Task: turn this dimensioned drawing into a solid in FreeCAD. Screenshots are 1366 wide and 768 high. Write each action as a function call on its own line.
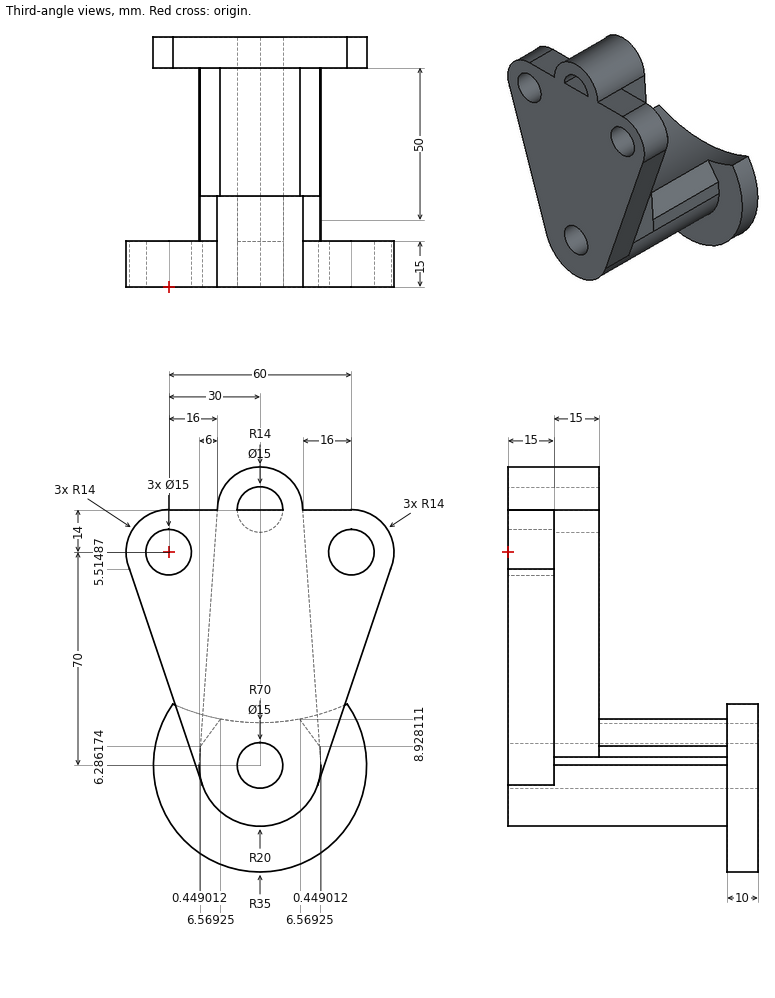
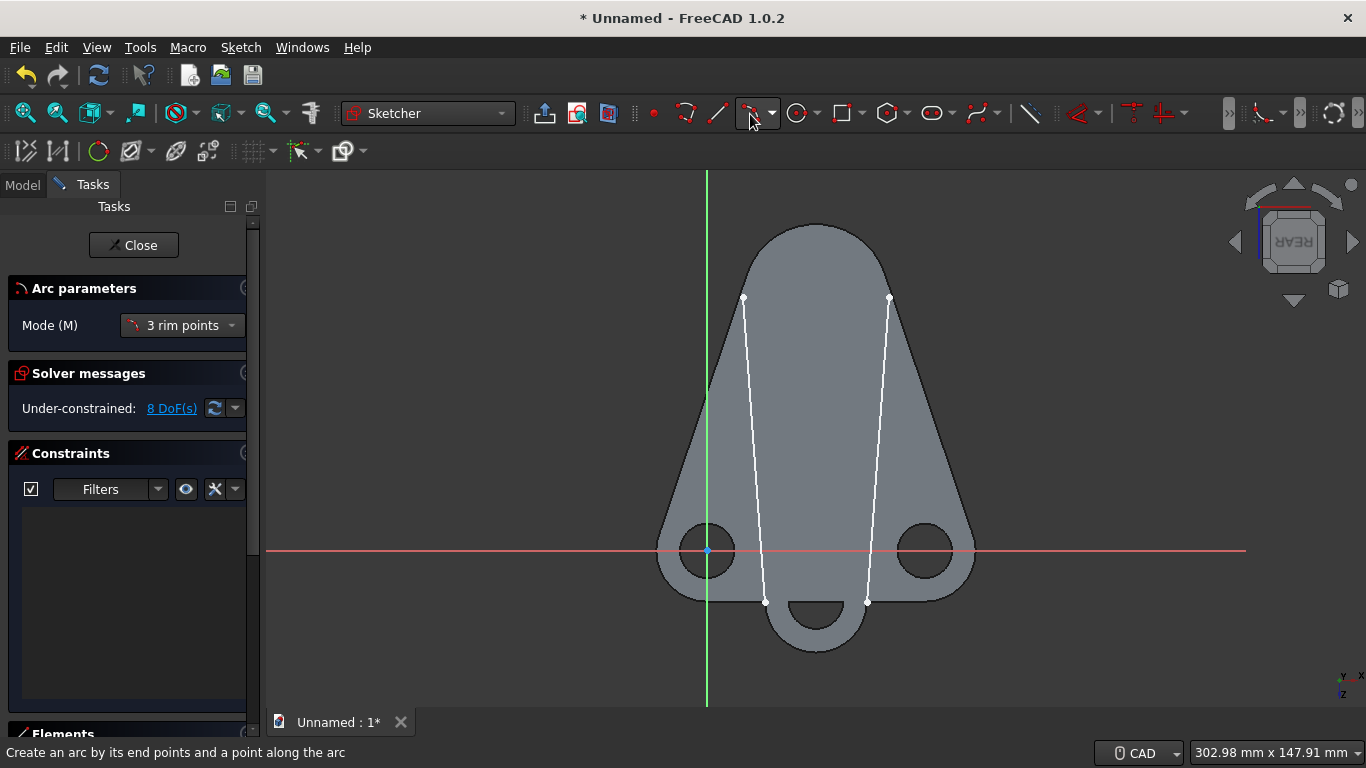
click(765, 603)
click(867, 603)
click(816, 653)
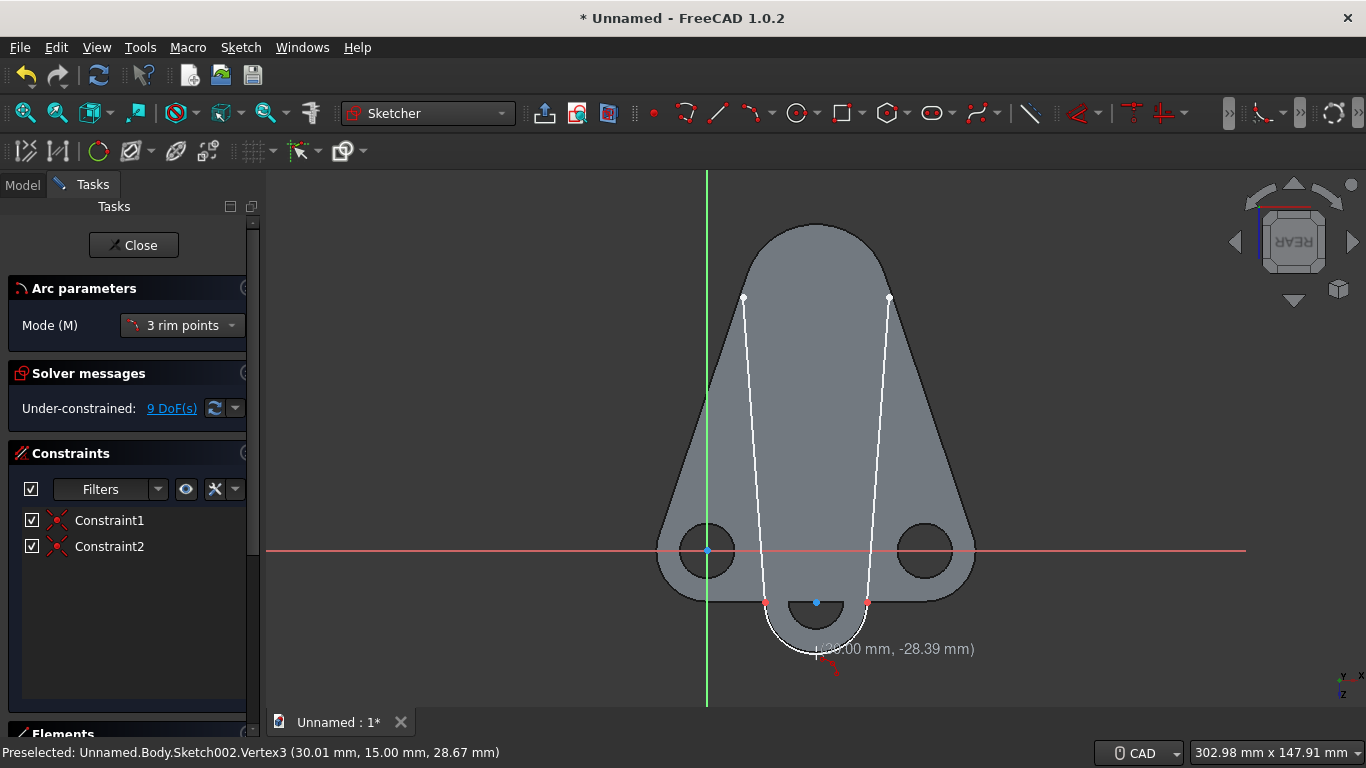
click(889, 298)
click(743, 298)
click(816, 224)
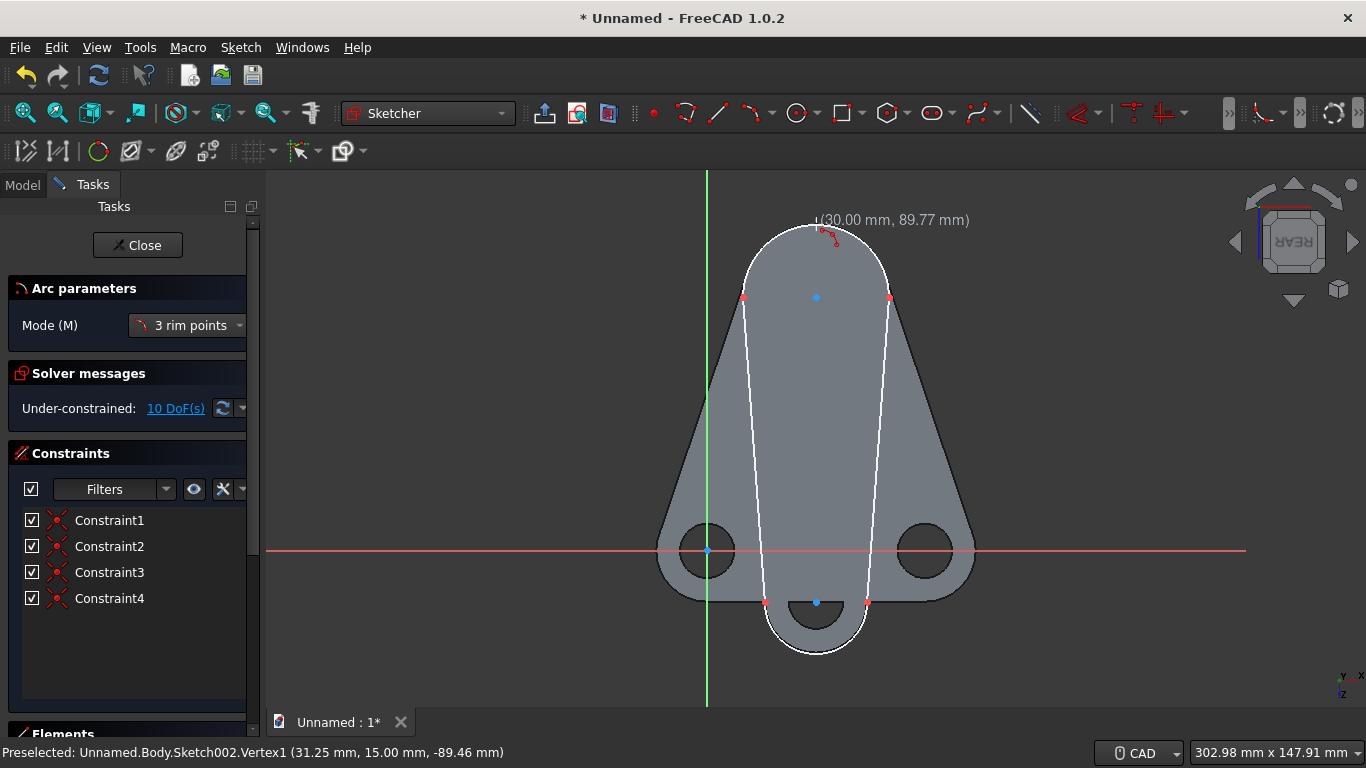
click(798, 114)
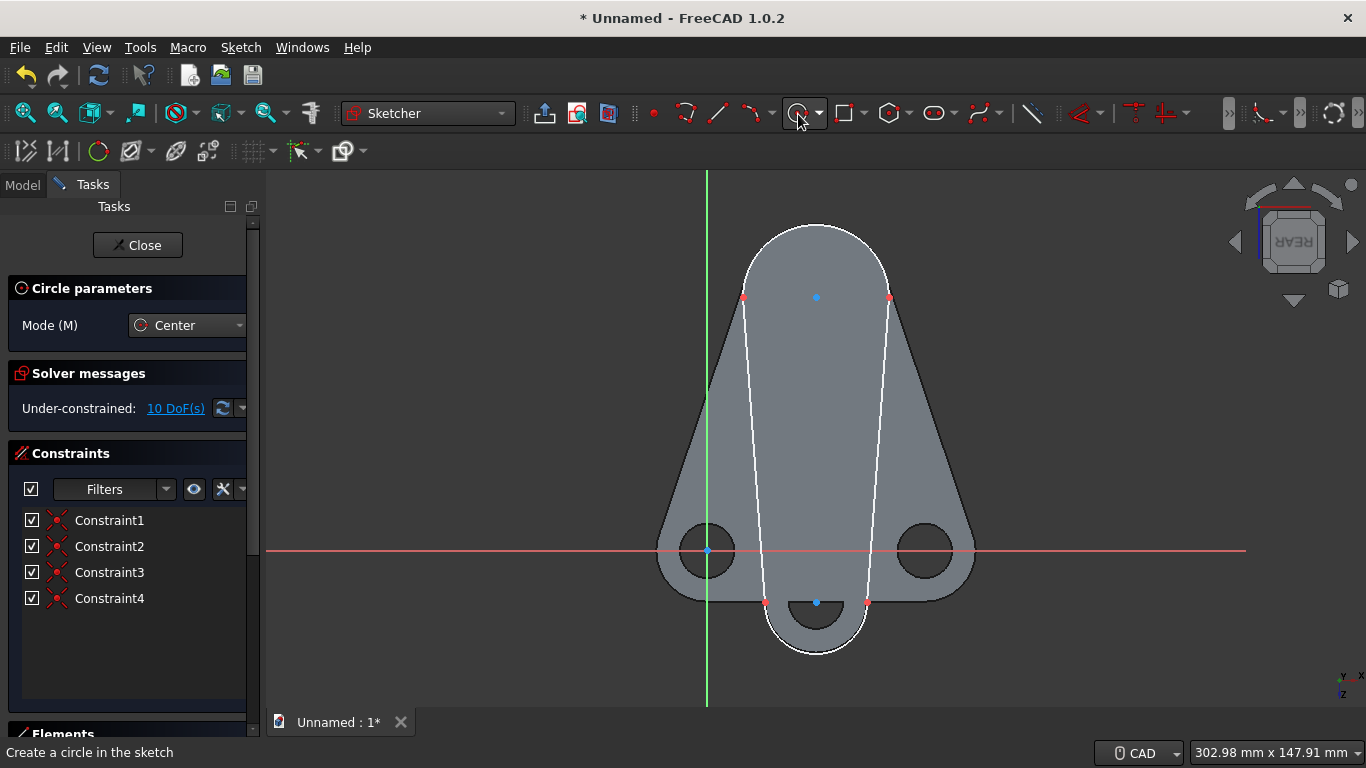
click(816, 602)
move(835, 583)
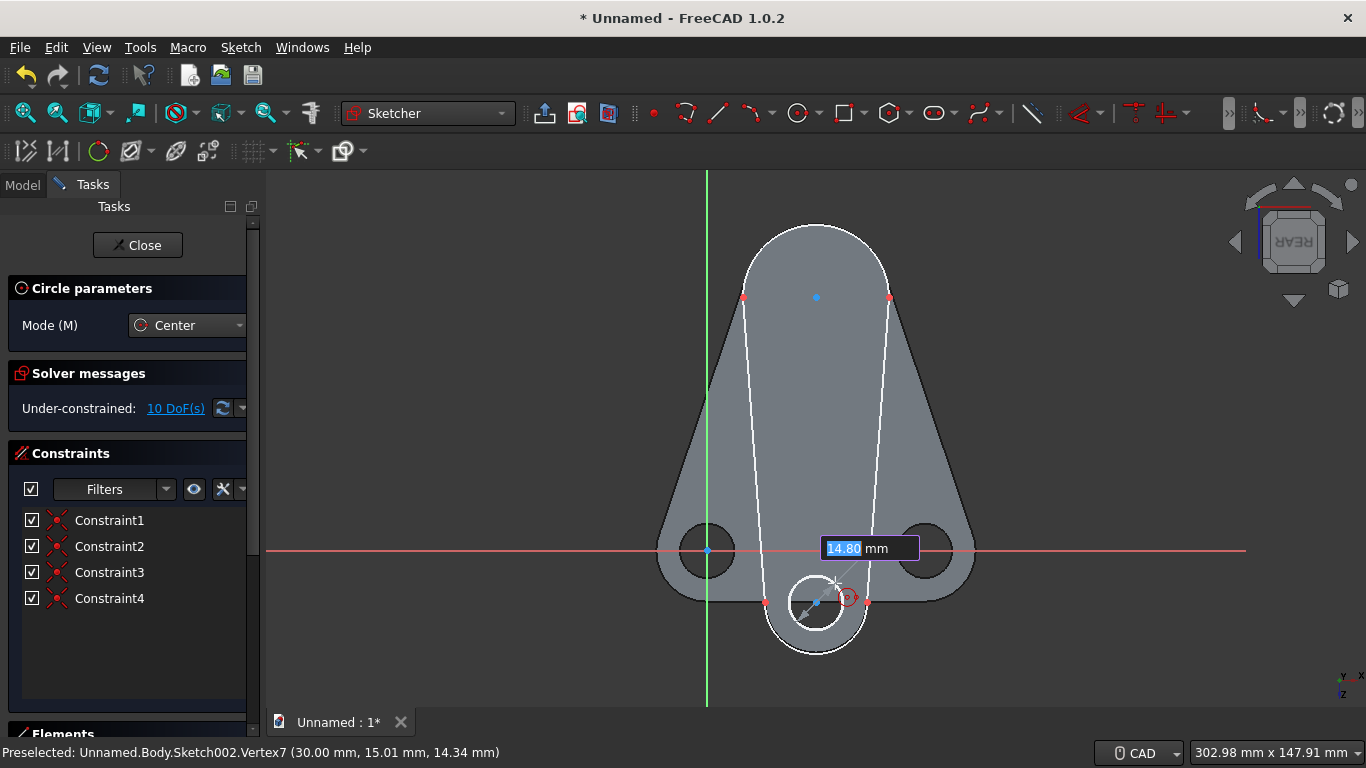
text(15)
key(Return)
key(Escape)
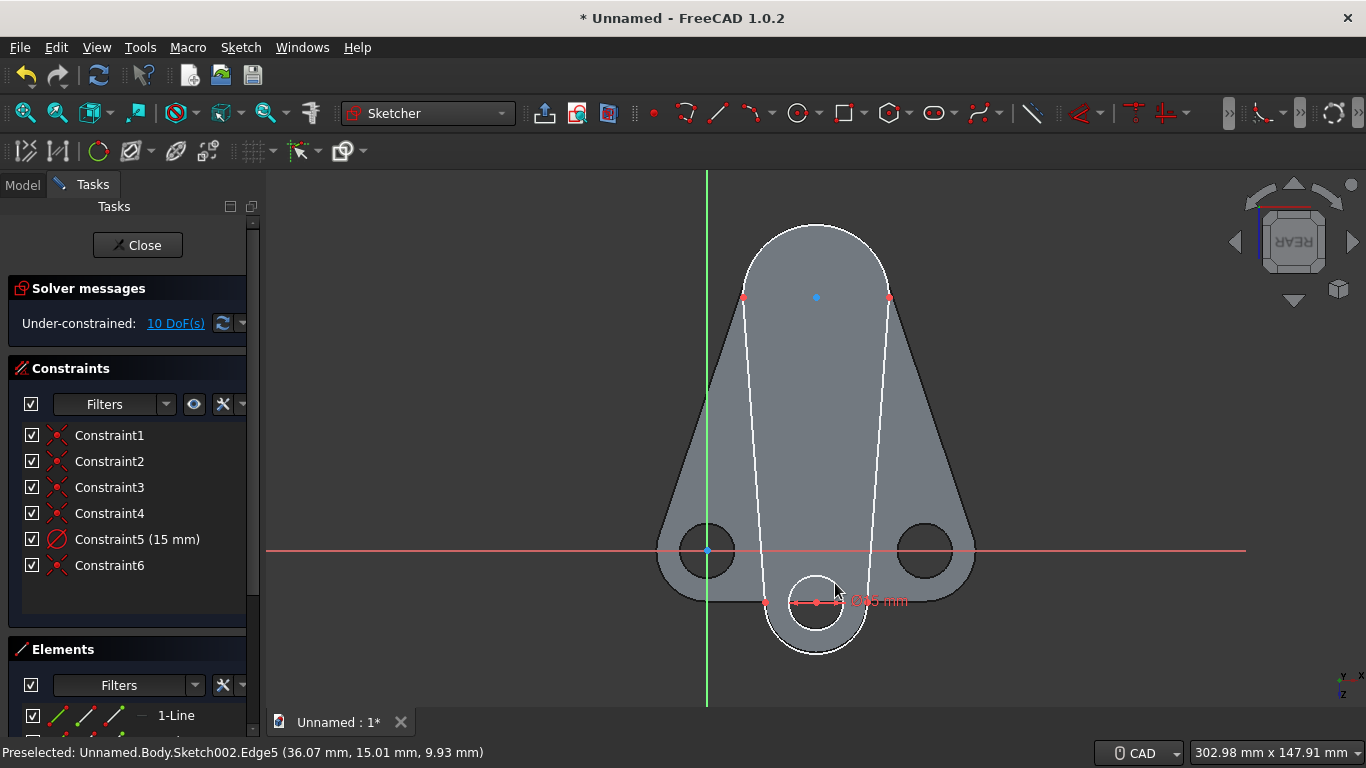
click(1080, 114)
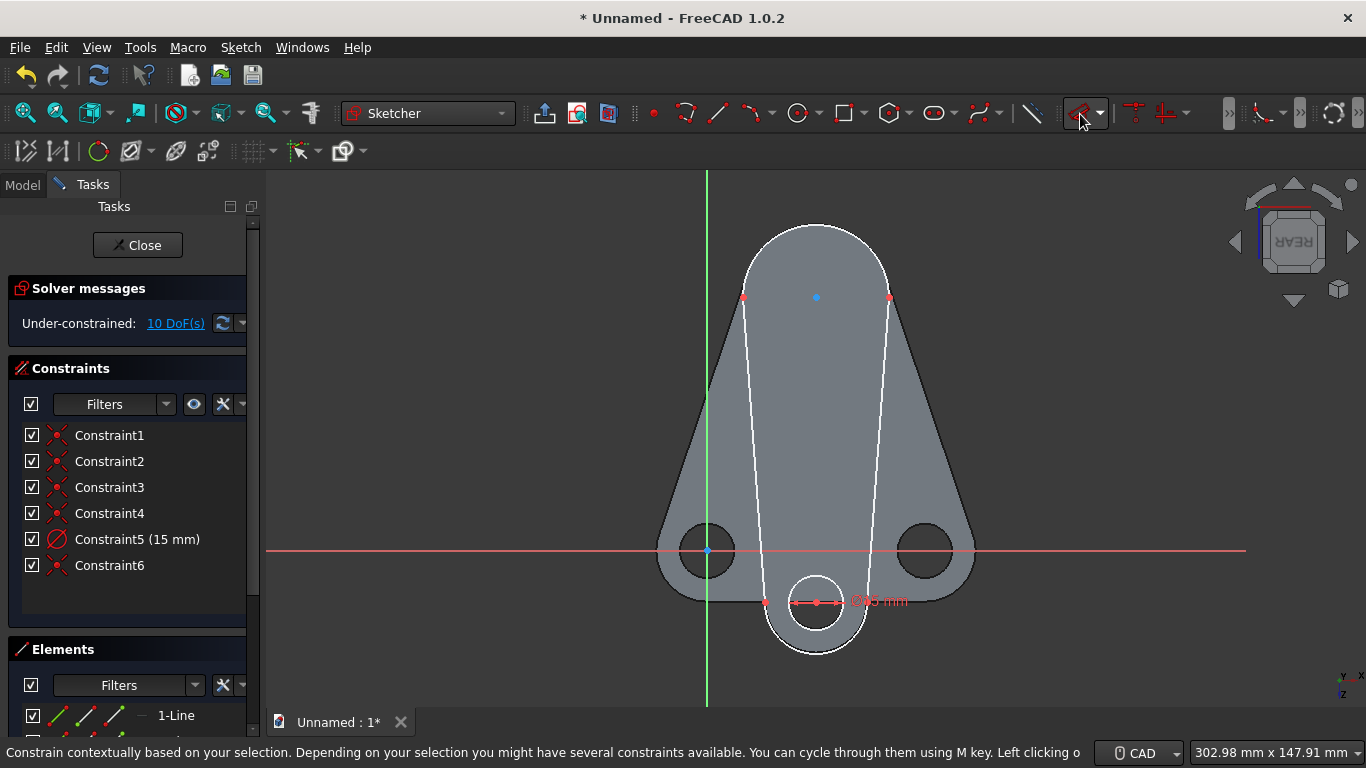
click(786, 644)
click(767, 670)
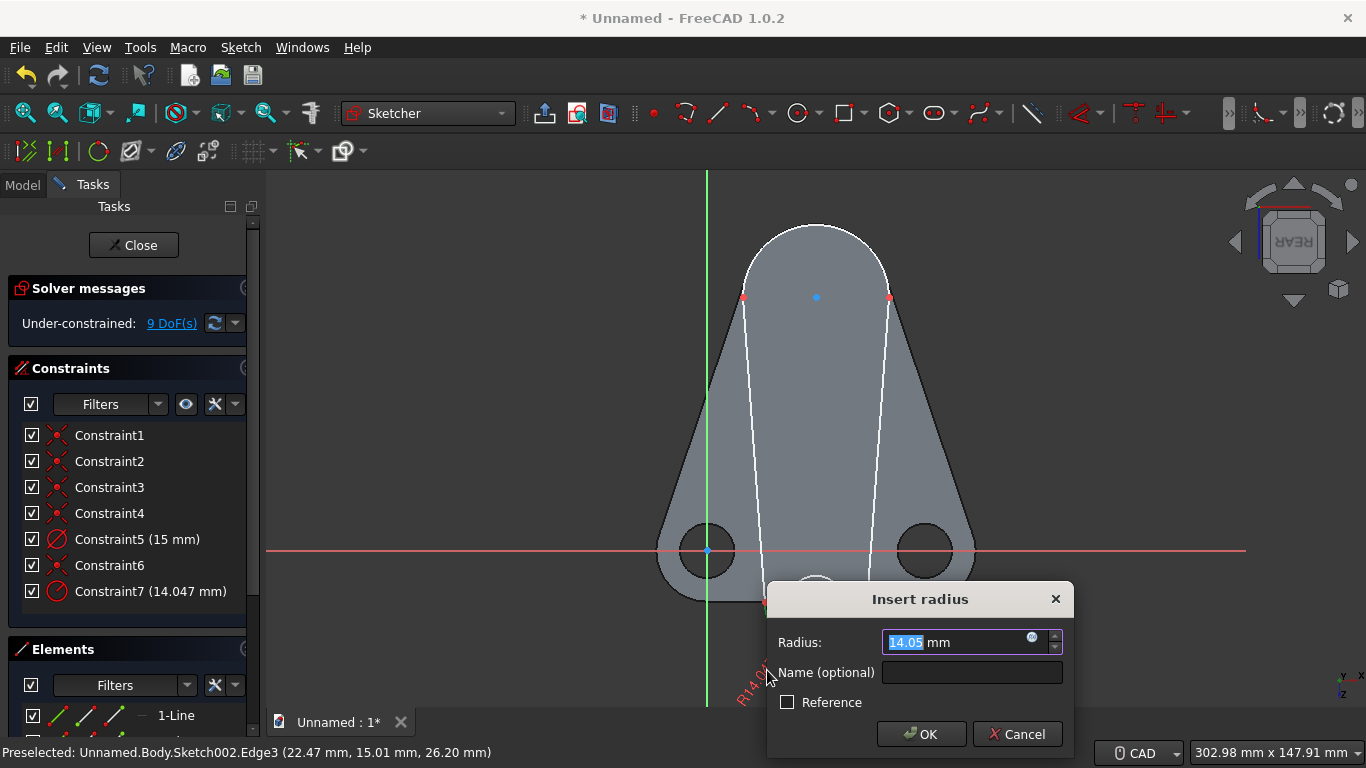
text(14)
key(Return)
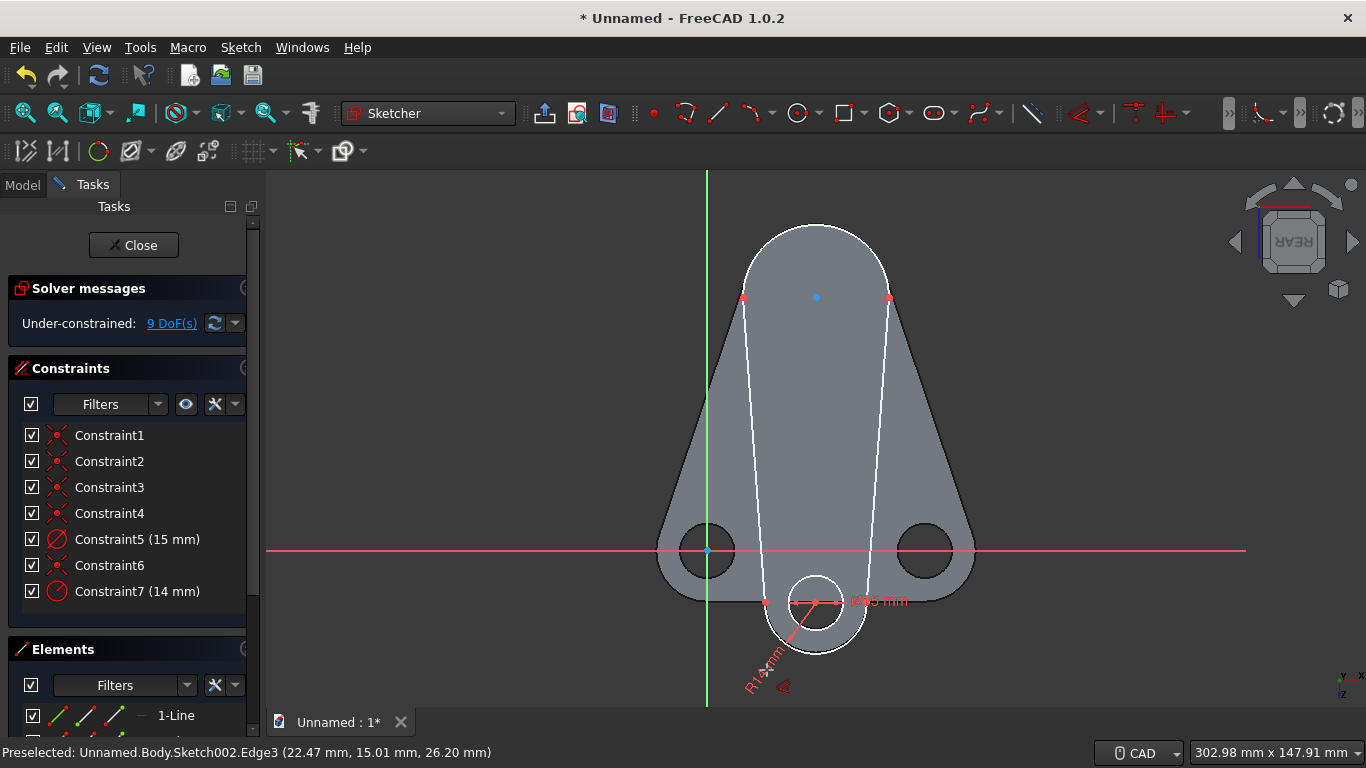
click(859, 239)
click(878, 213)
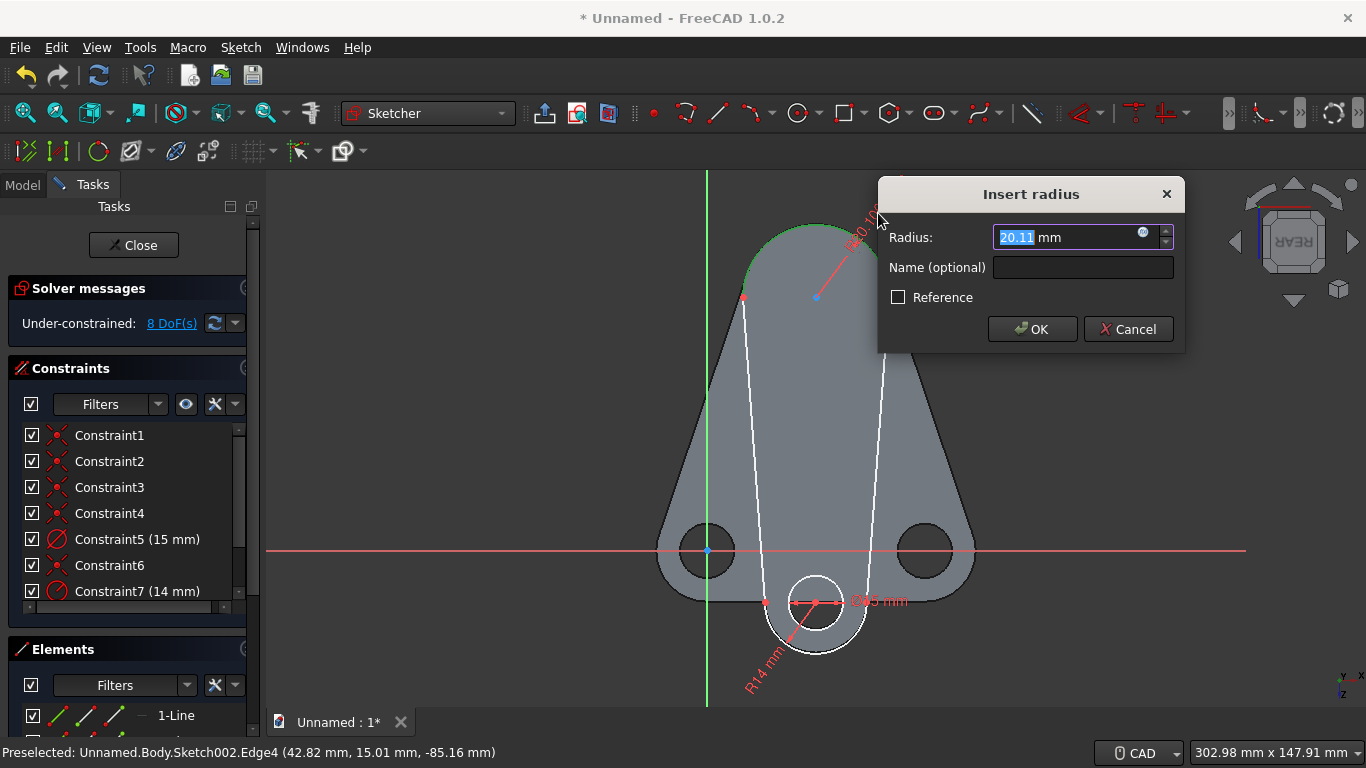
text(20)
key(Return)